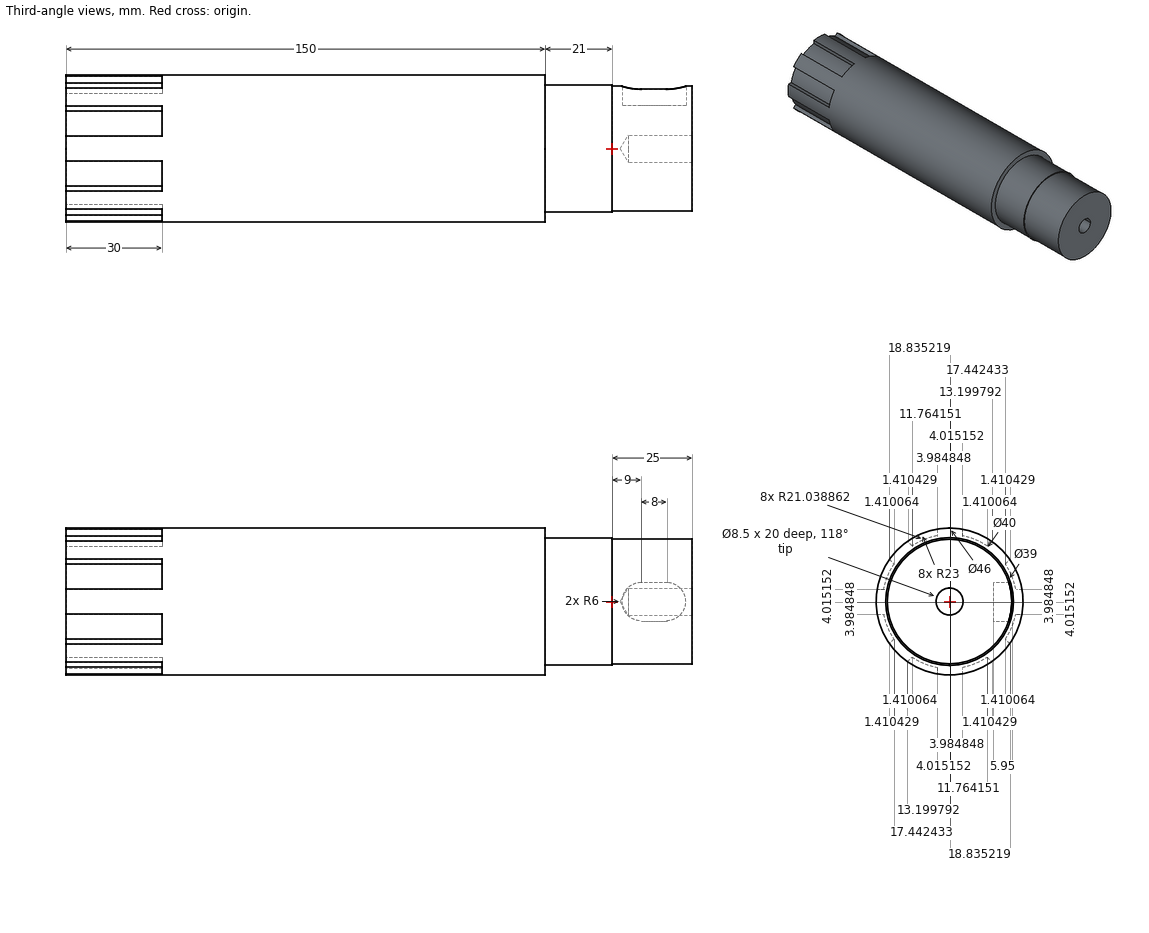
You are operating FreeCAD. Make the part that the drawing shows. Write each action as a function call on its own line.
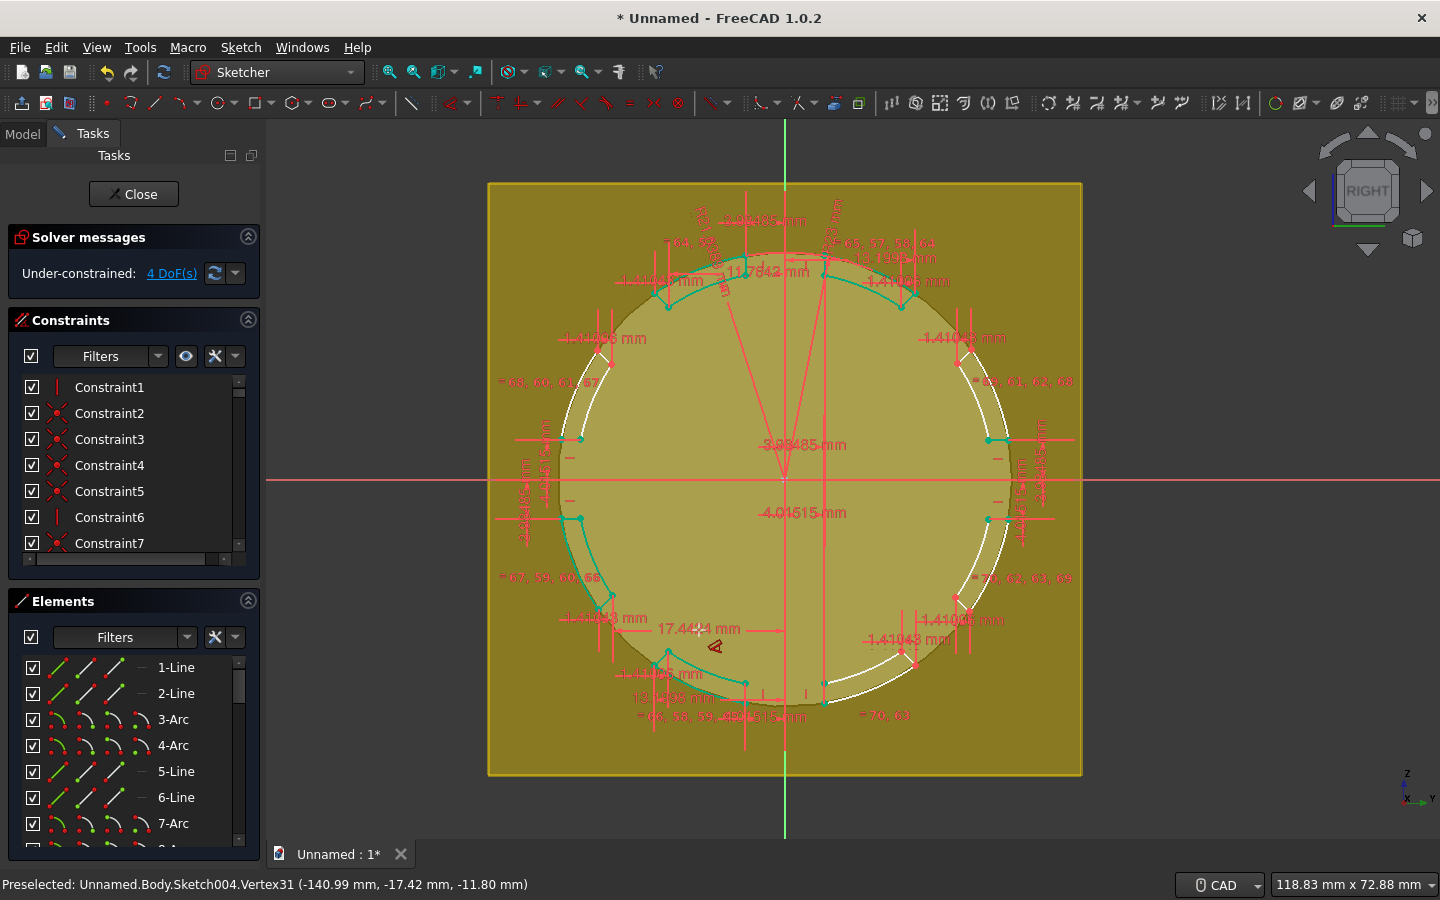
click(598, 351)
click(691, 317)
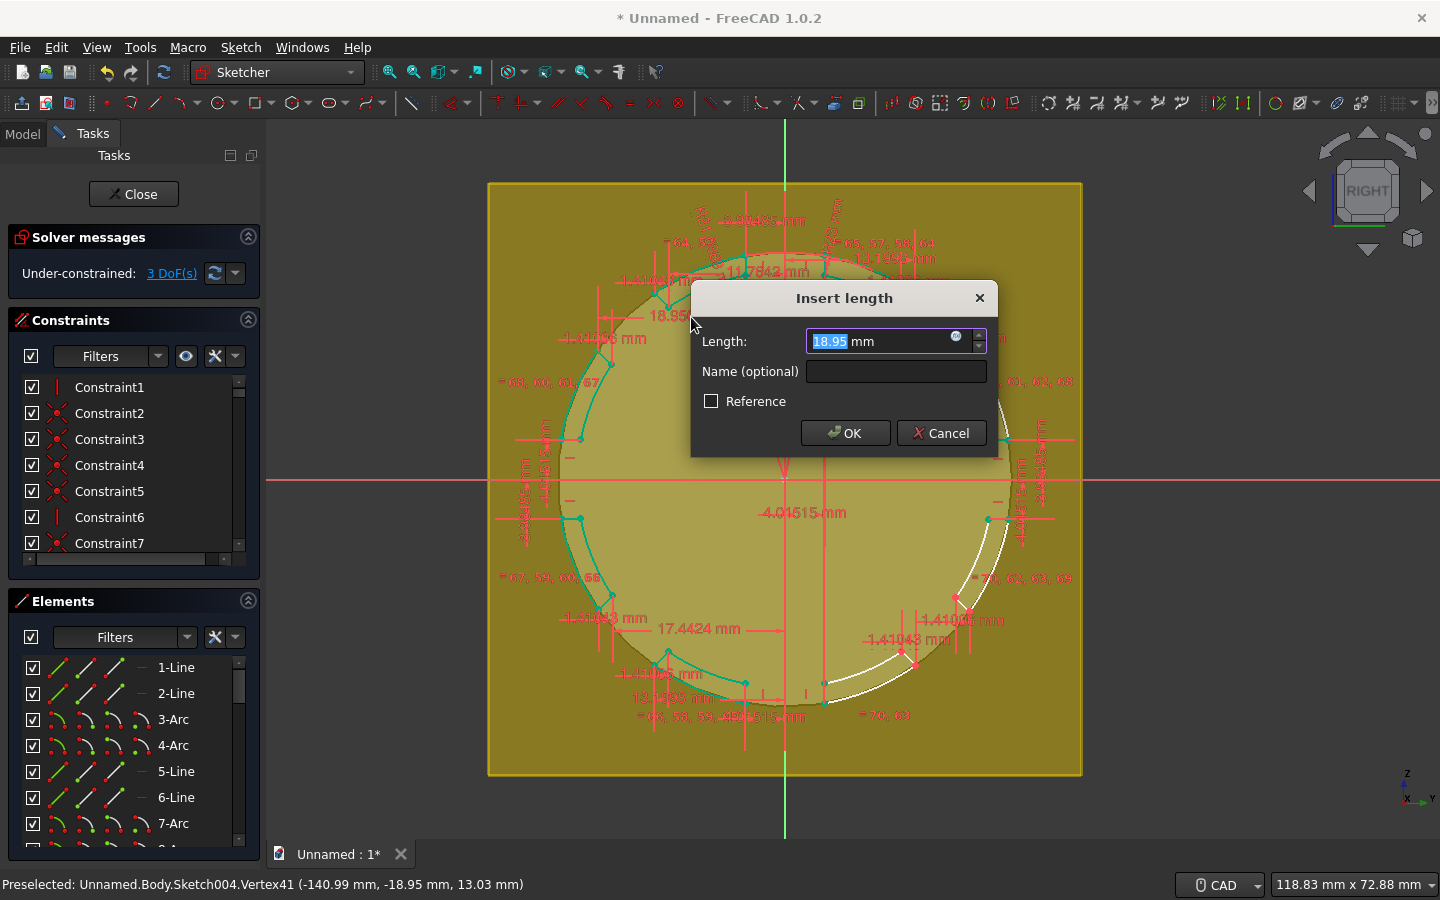
text(18.835219)
key(Return)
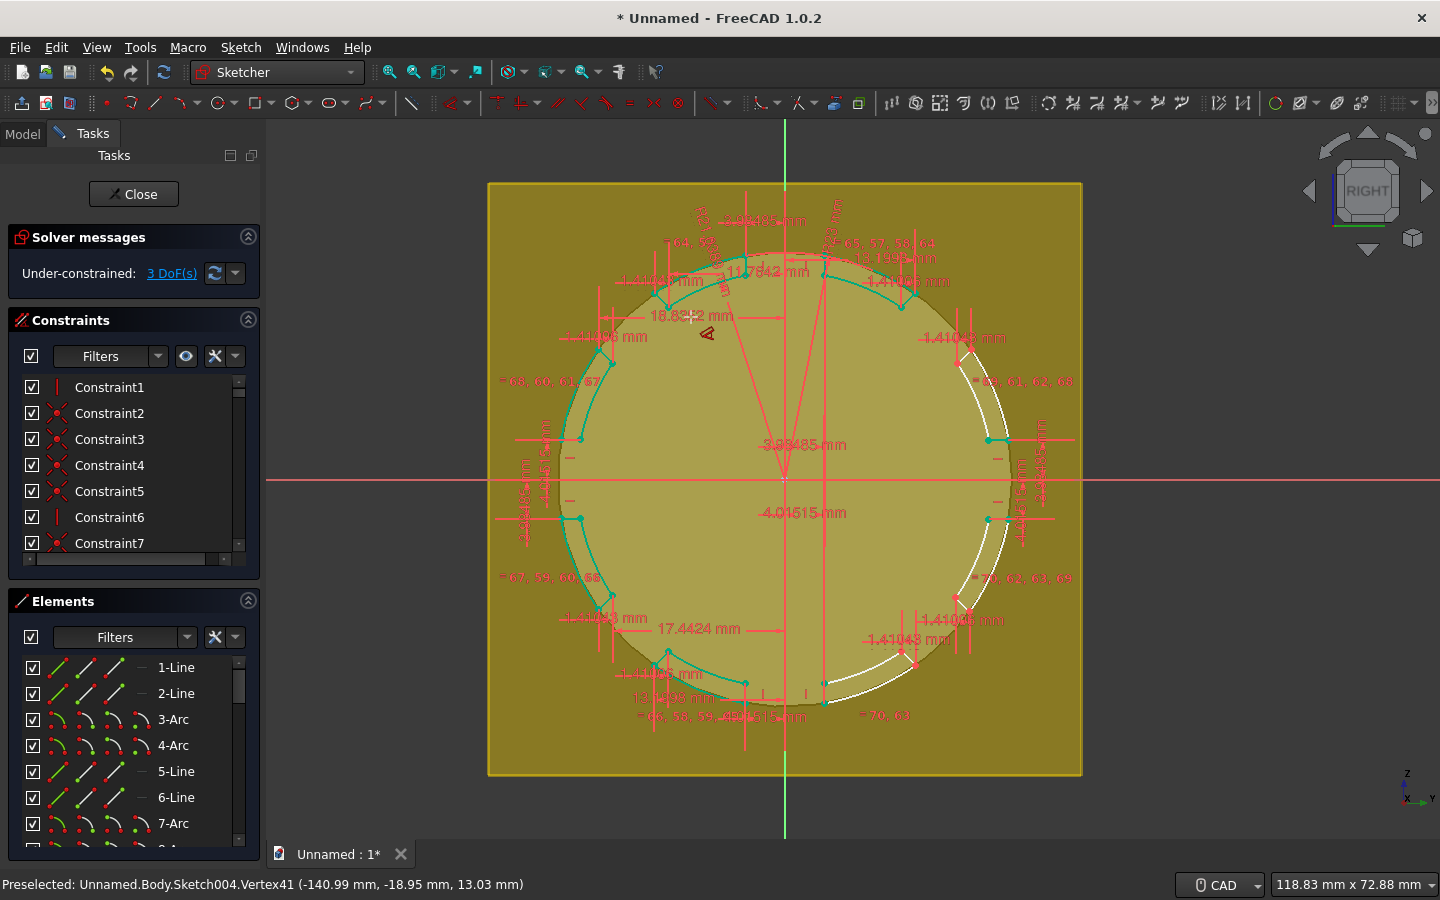
click(957, 364)
click(871, 330)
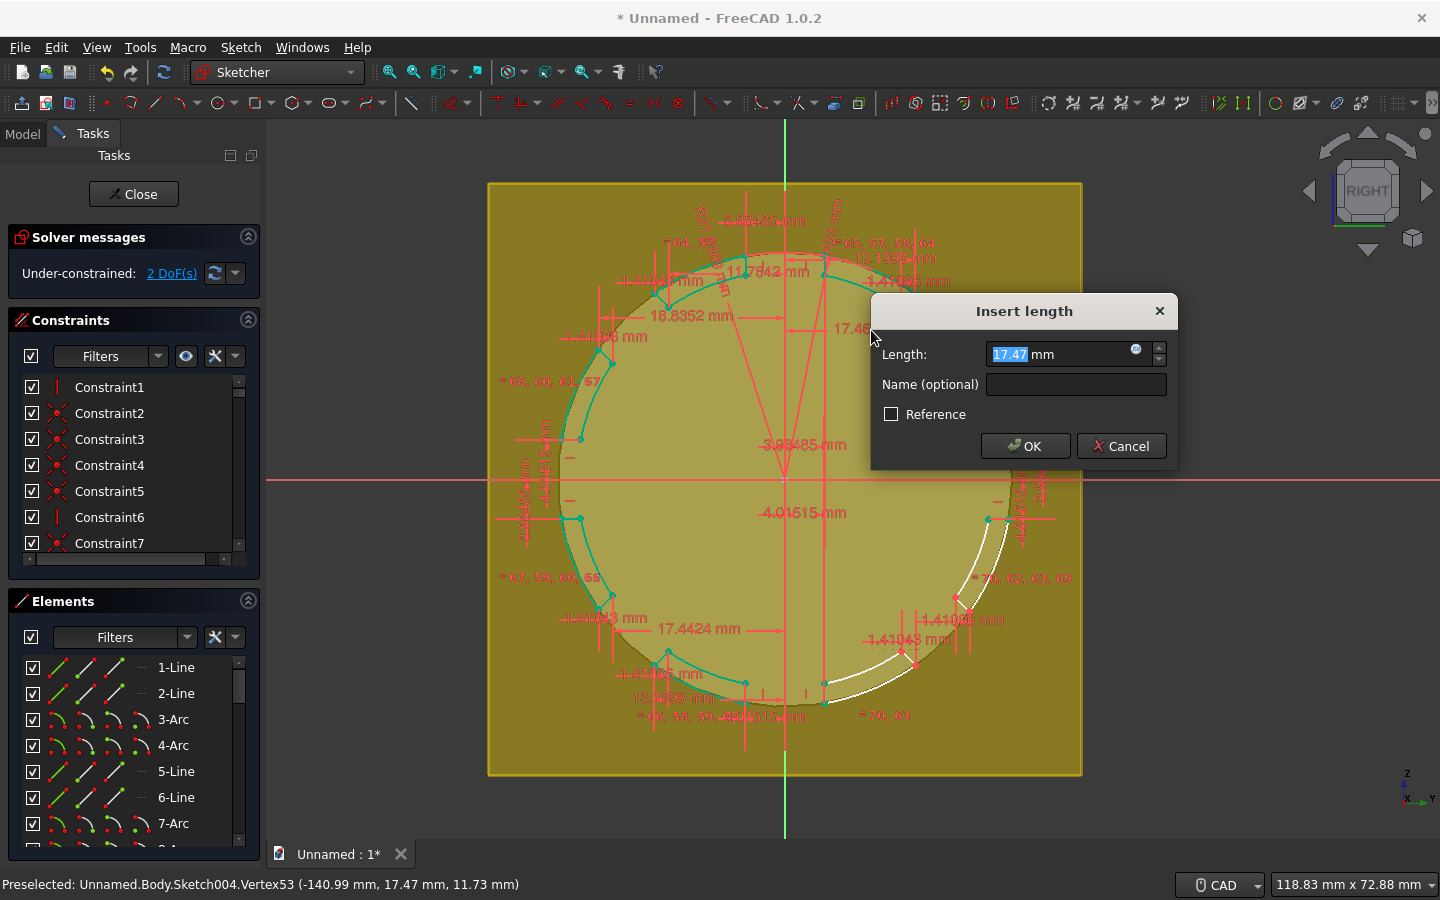
text(17.442433)
key(Return)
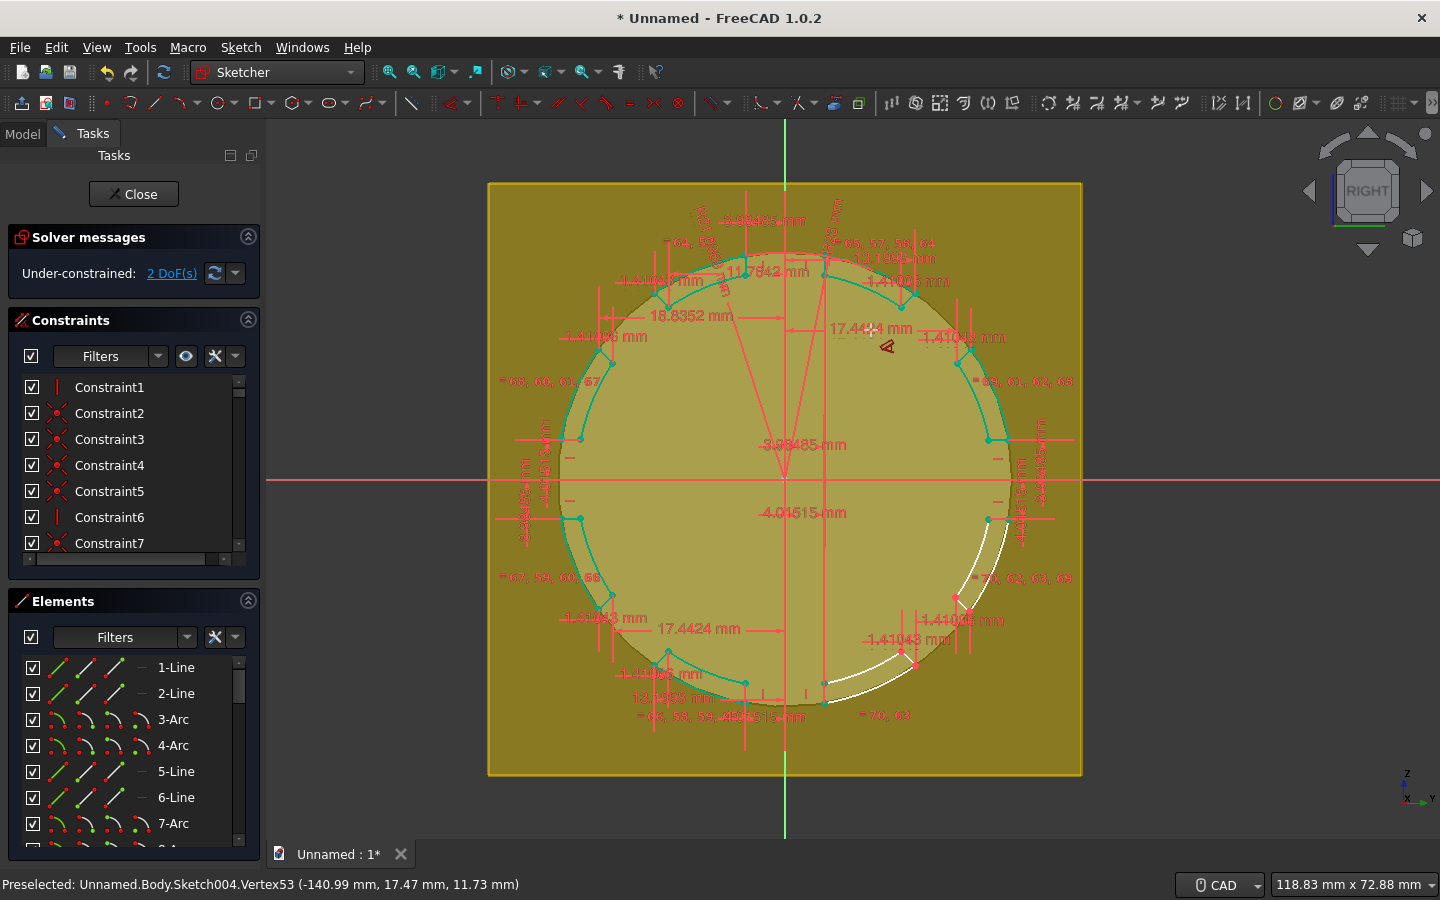
click(970, 612)
click(835, 646)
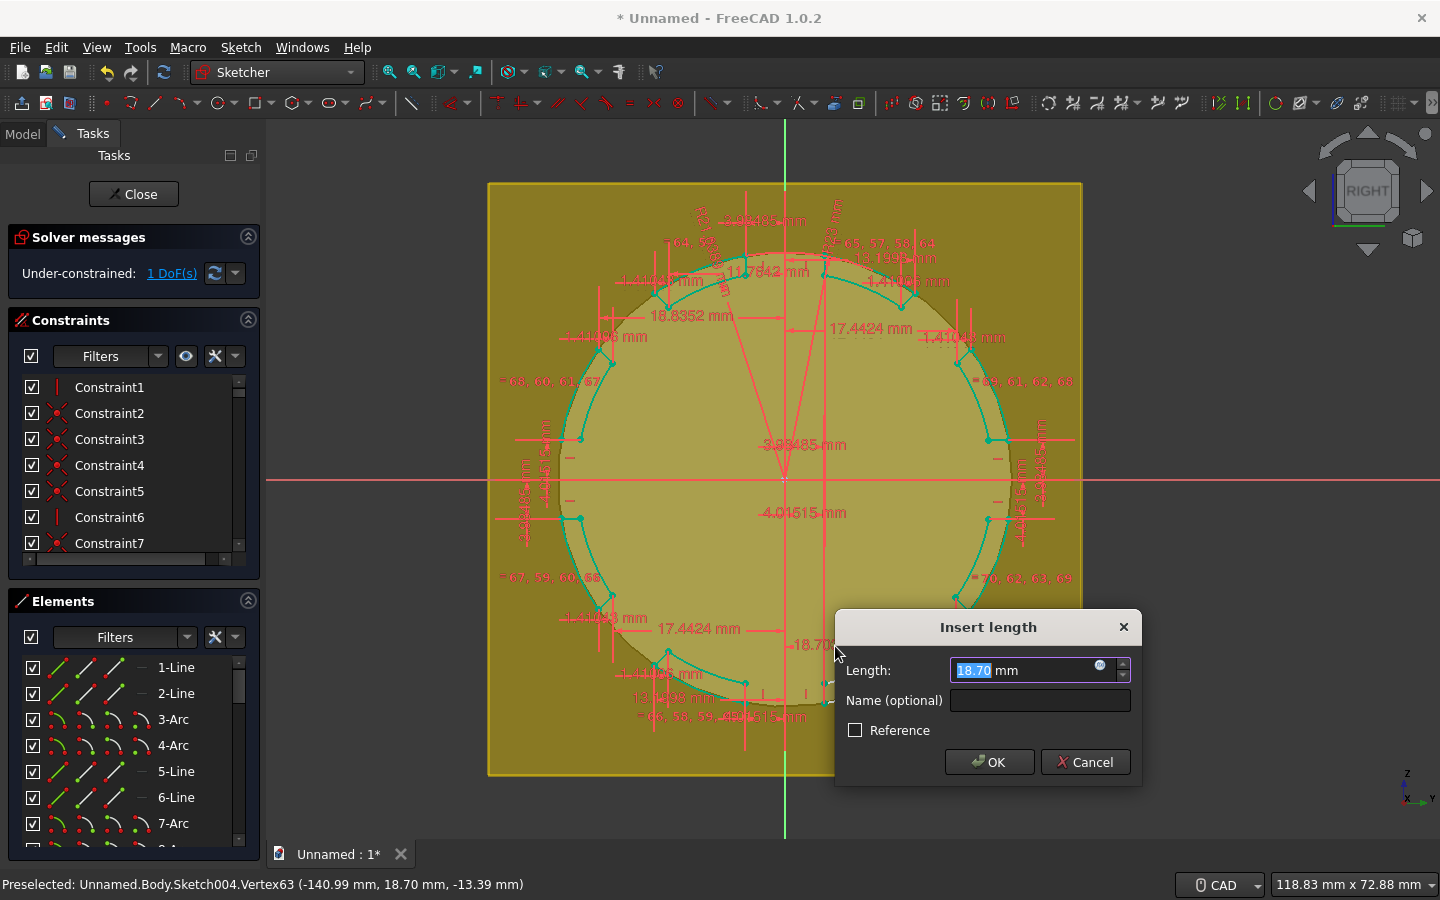
text(18.835219)
key(Return)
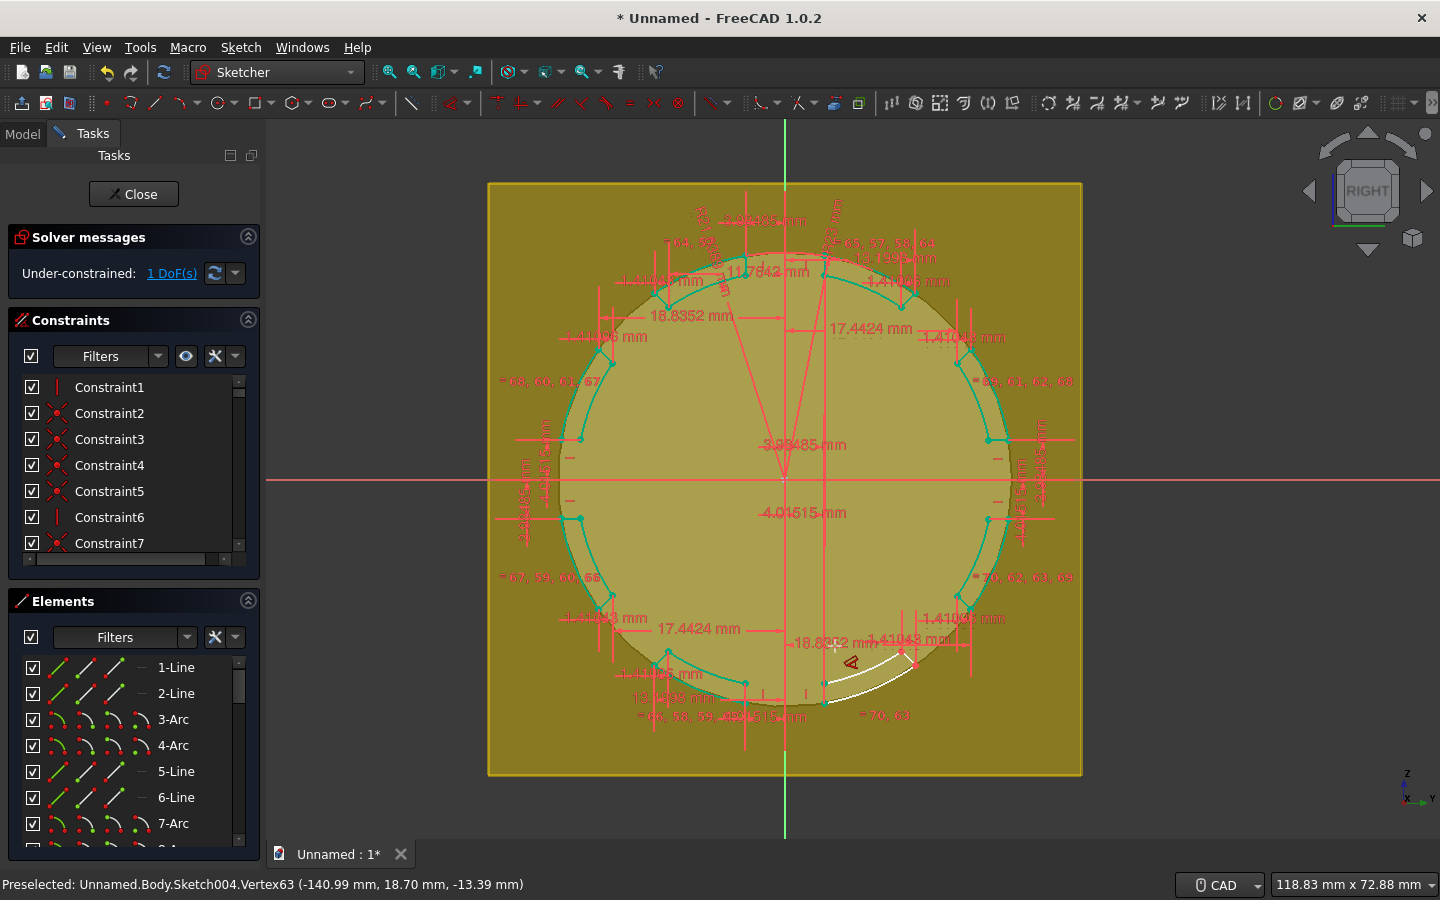
click(902, 651)
click(802, 685)